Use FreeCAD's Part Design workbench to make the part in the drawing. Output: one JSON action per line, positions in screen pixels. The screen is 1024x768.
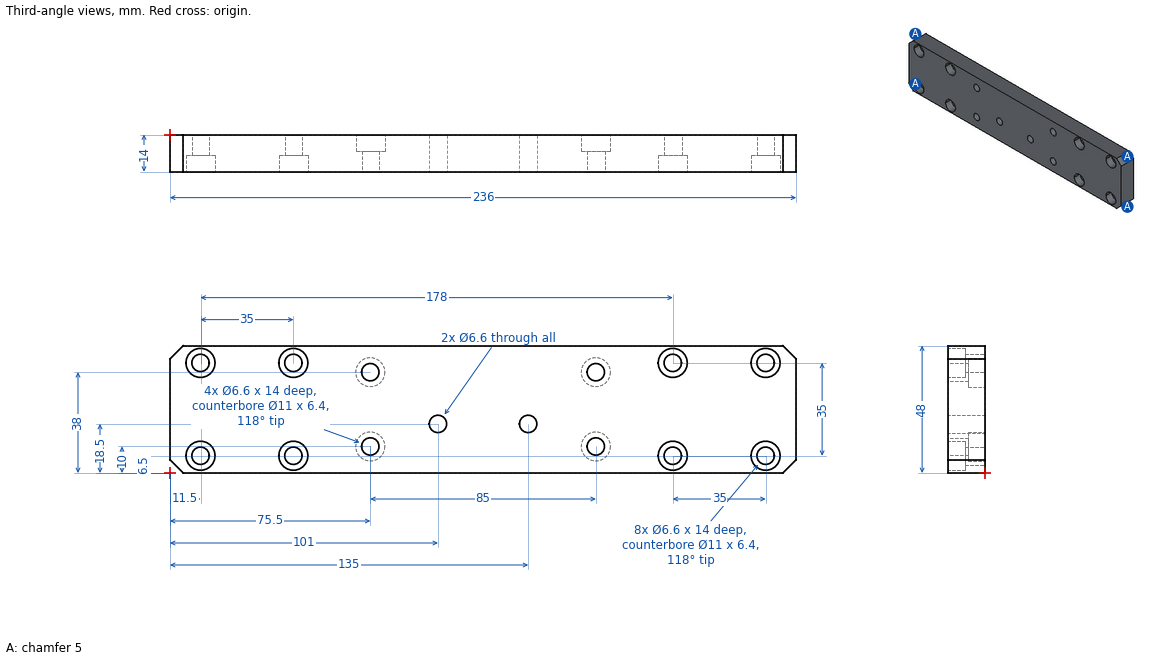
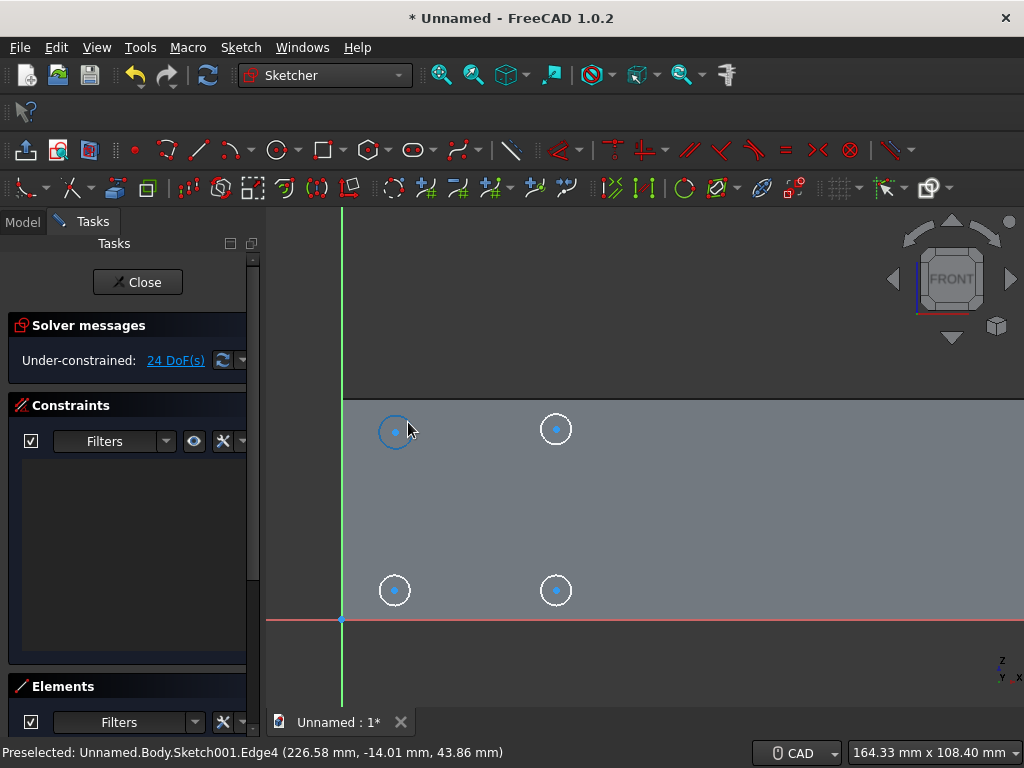
{"action": "left_click", "coordinate": [408, 420]}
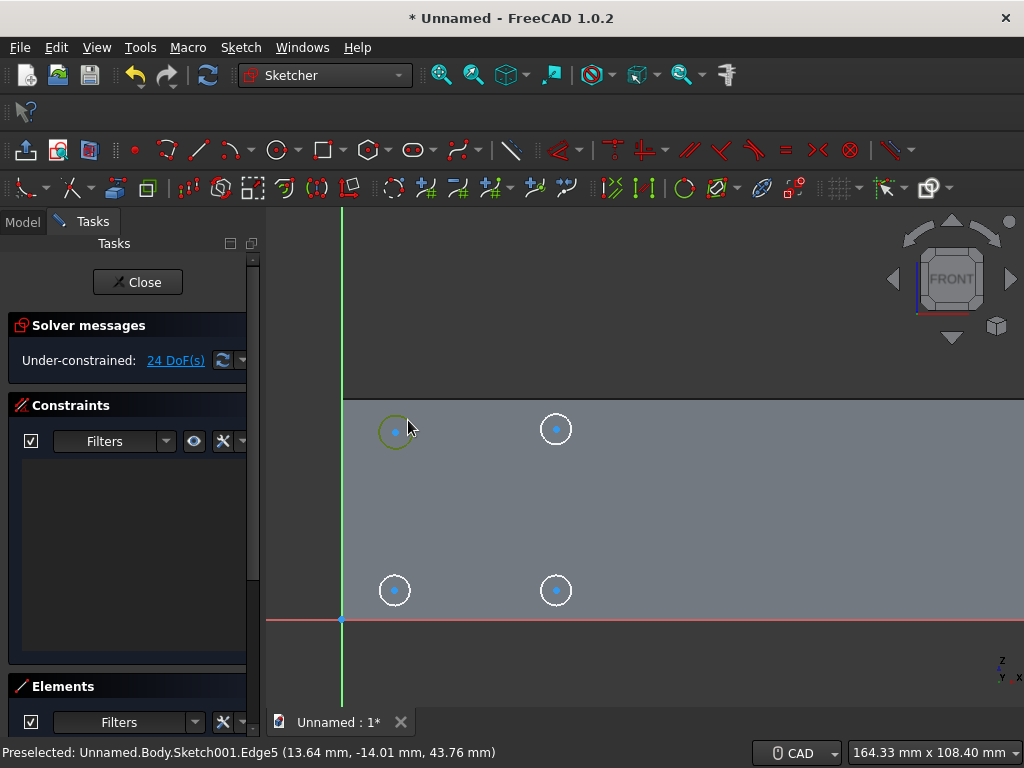
{"action": "left_click", "coordinate": [567, 419]}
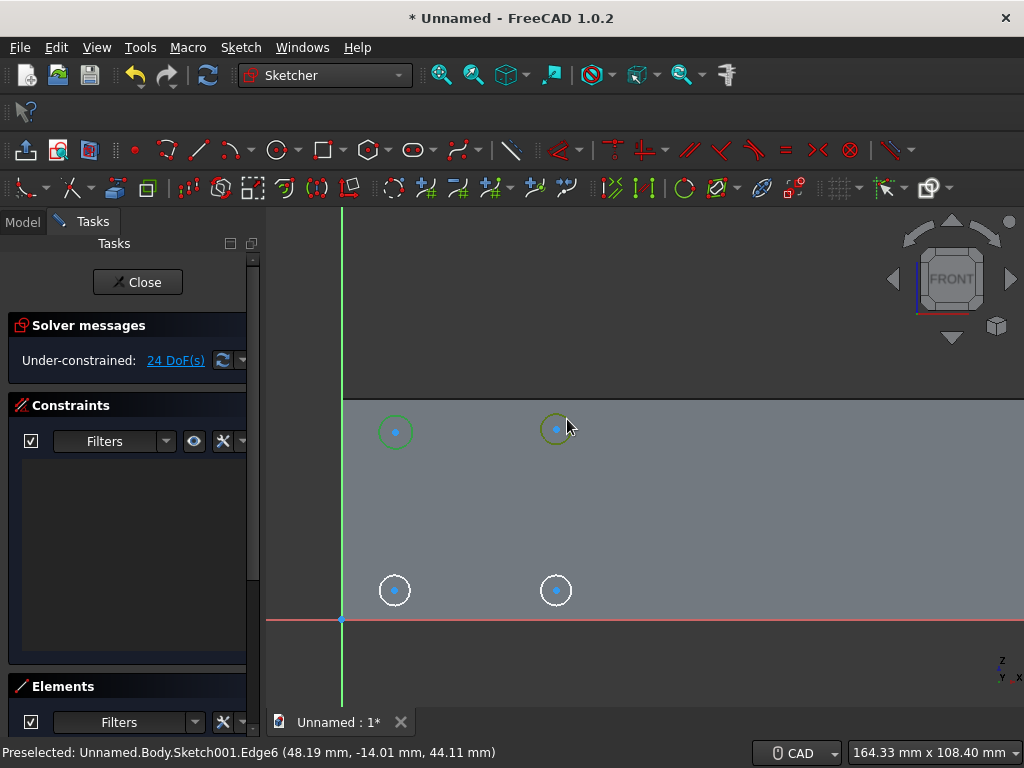
{"action": "left_click", "coordinate": [567, 580]}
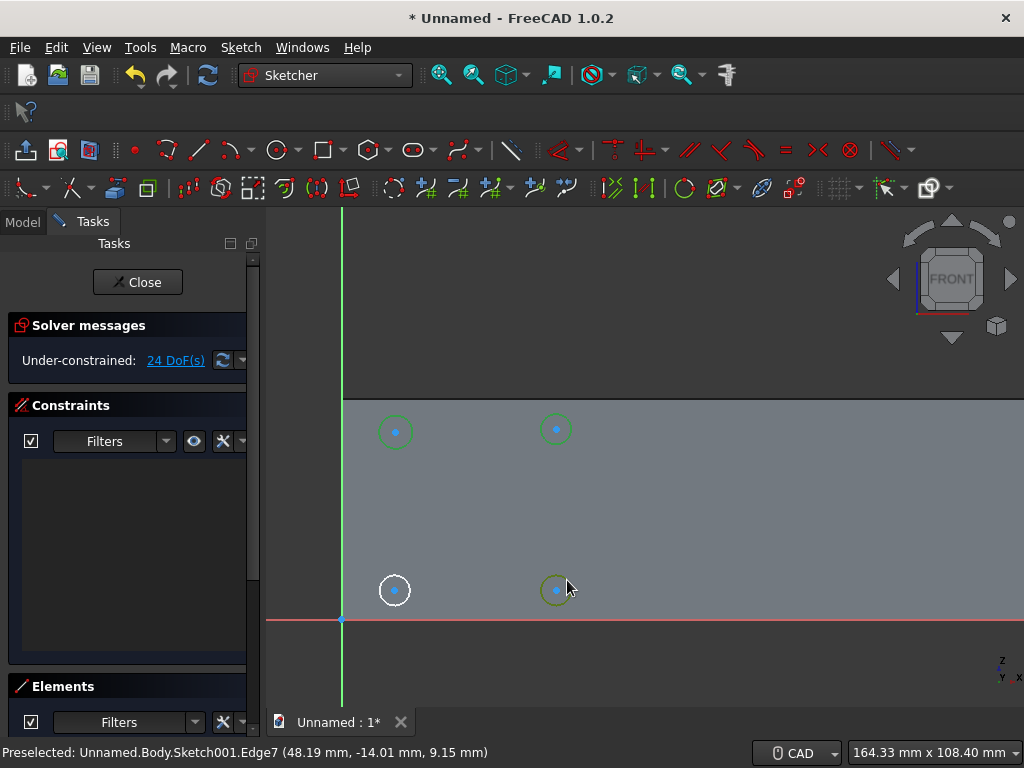
{"action": "left_click", "coordinate": [405, 580]}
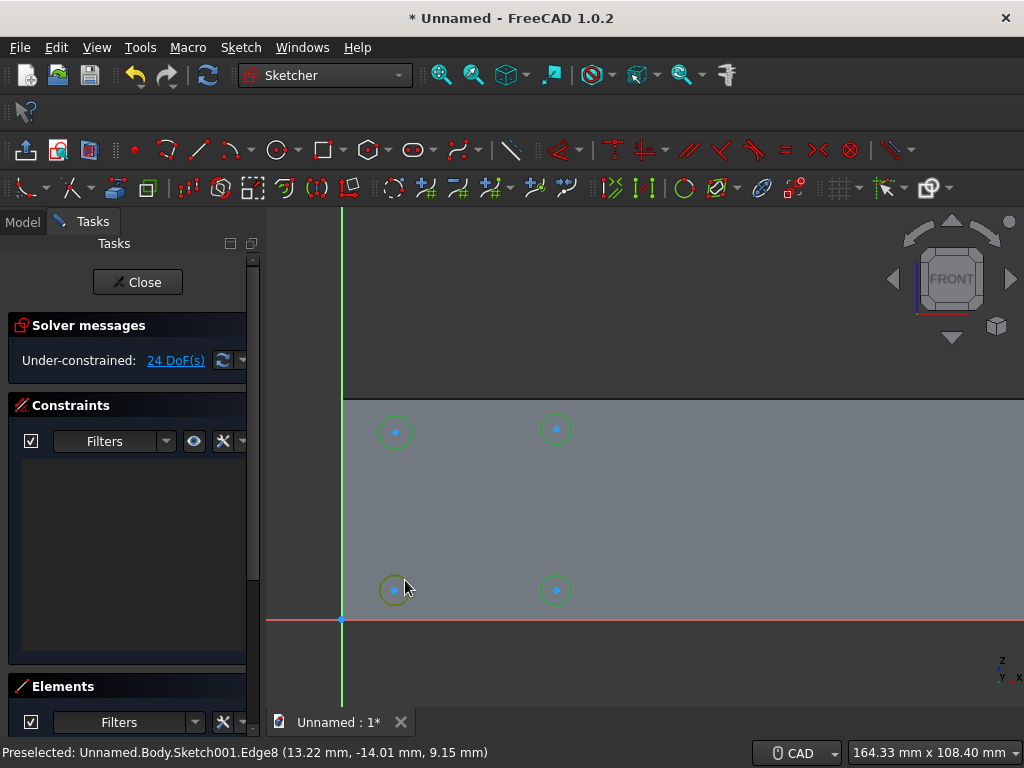
{"action": "left_click", "coordinate": [786, 150]}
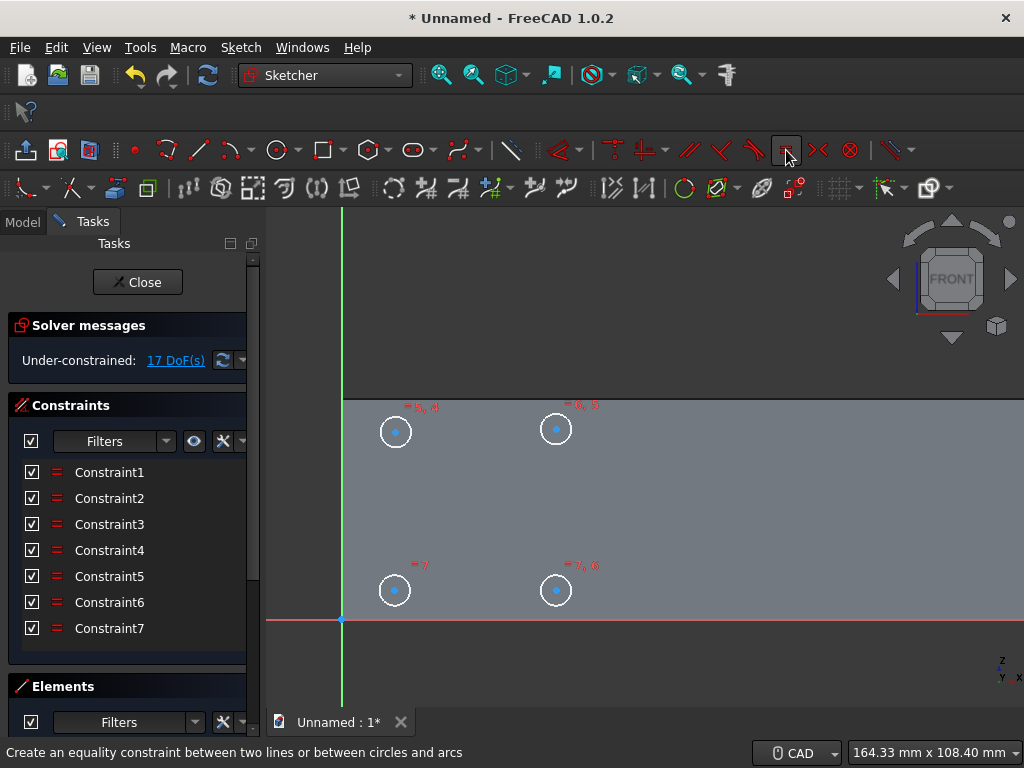
{"action": "scroll", "coordinate": [407, 422], "scroll_direction": "down", "scroll_amount": 5}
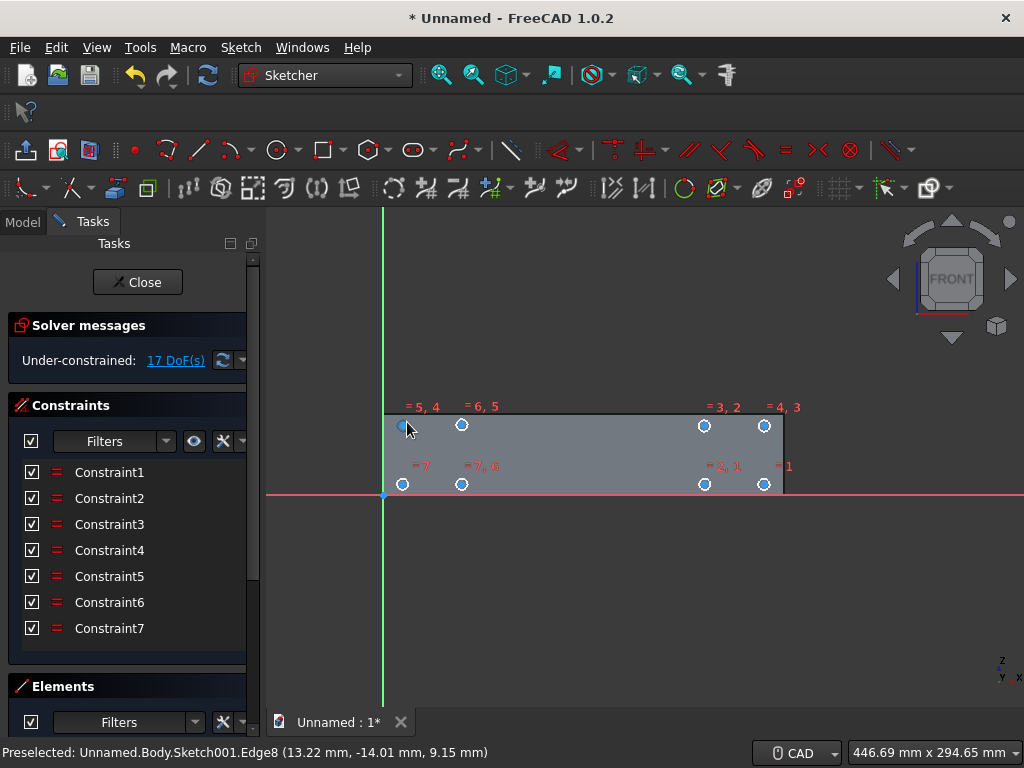
{"action": "left_click", "coordinate": [764, 484]}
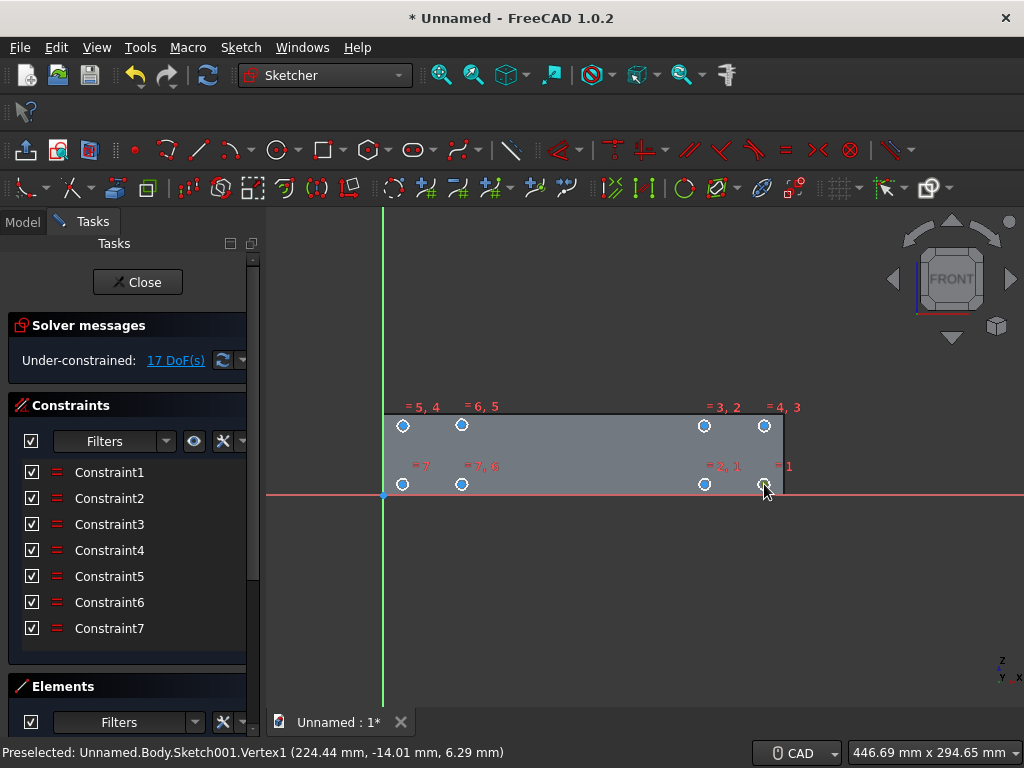
{"action": "left_click", "coordinate": [705, 484]}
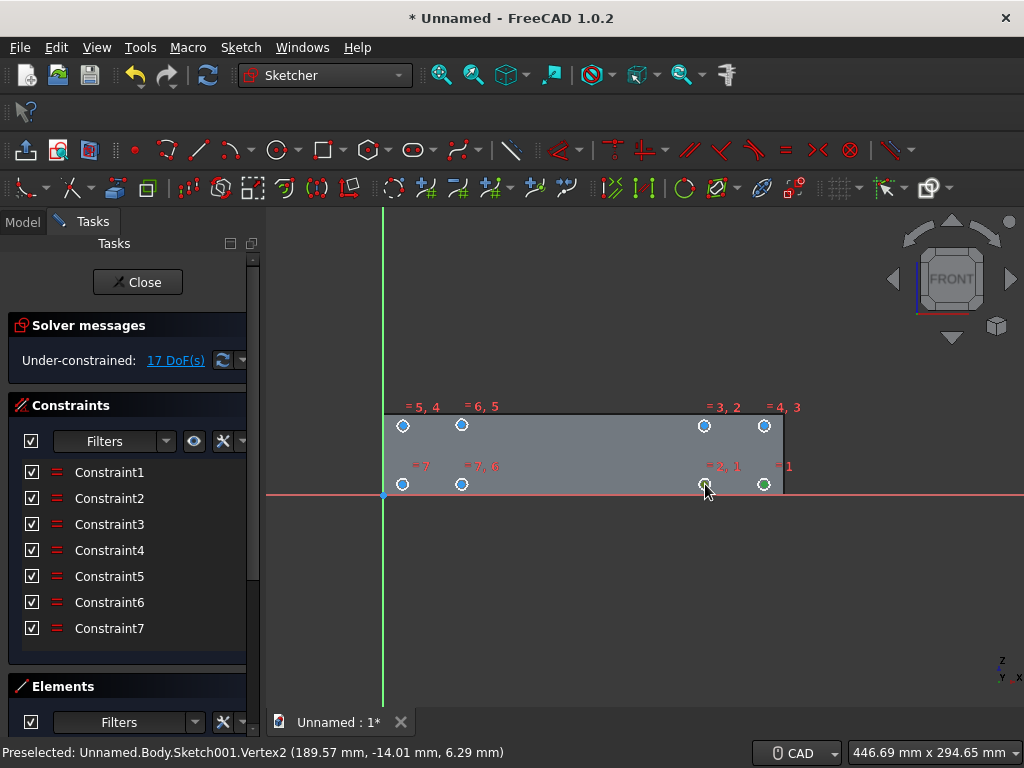
{"action": "left_click", "coordinate": [668, 150]}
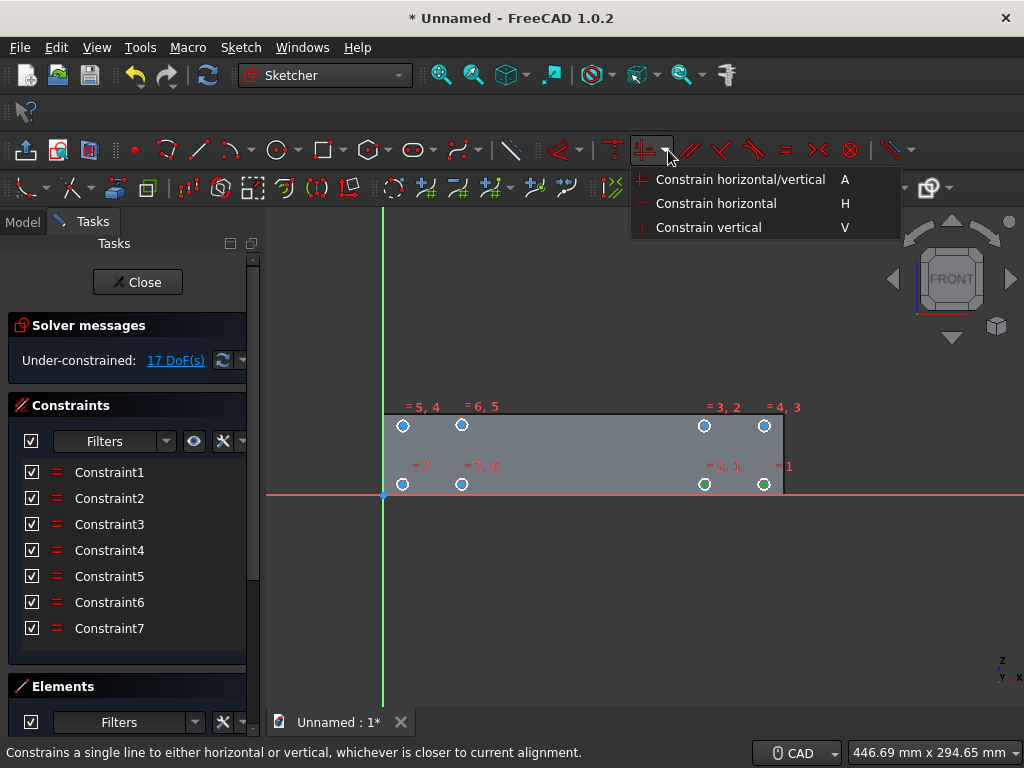
{"action": "left_click", "coordinate": [766, 203]}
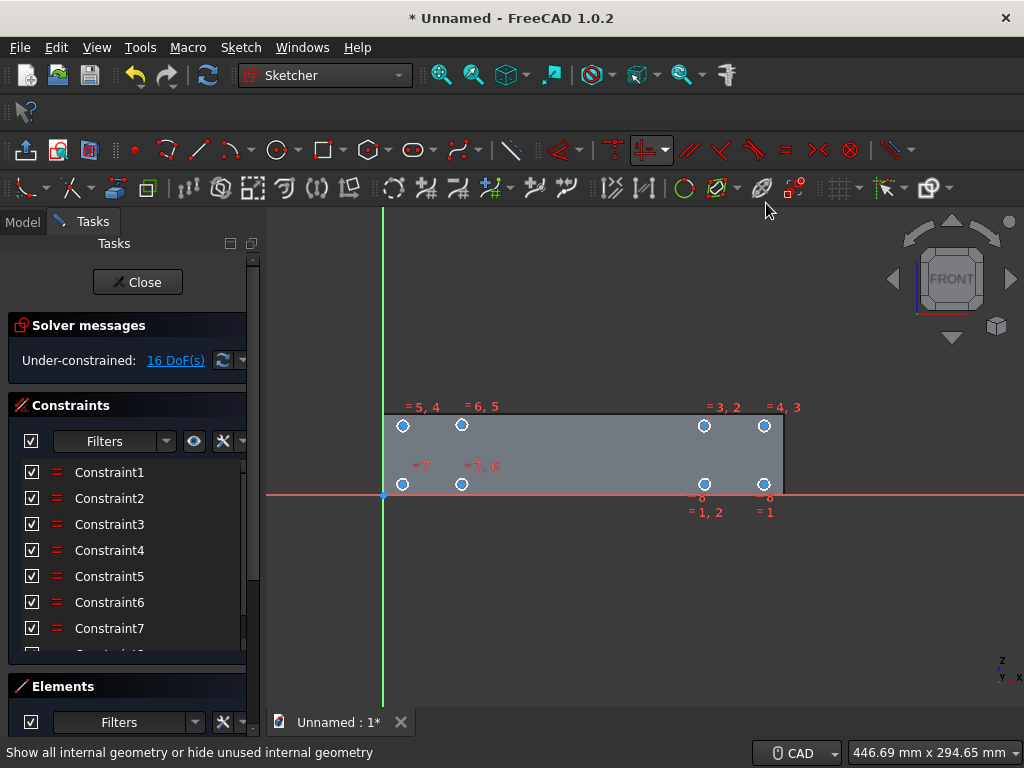
{"action": "left_click", "coordinate": [705, 484]}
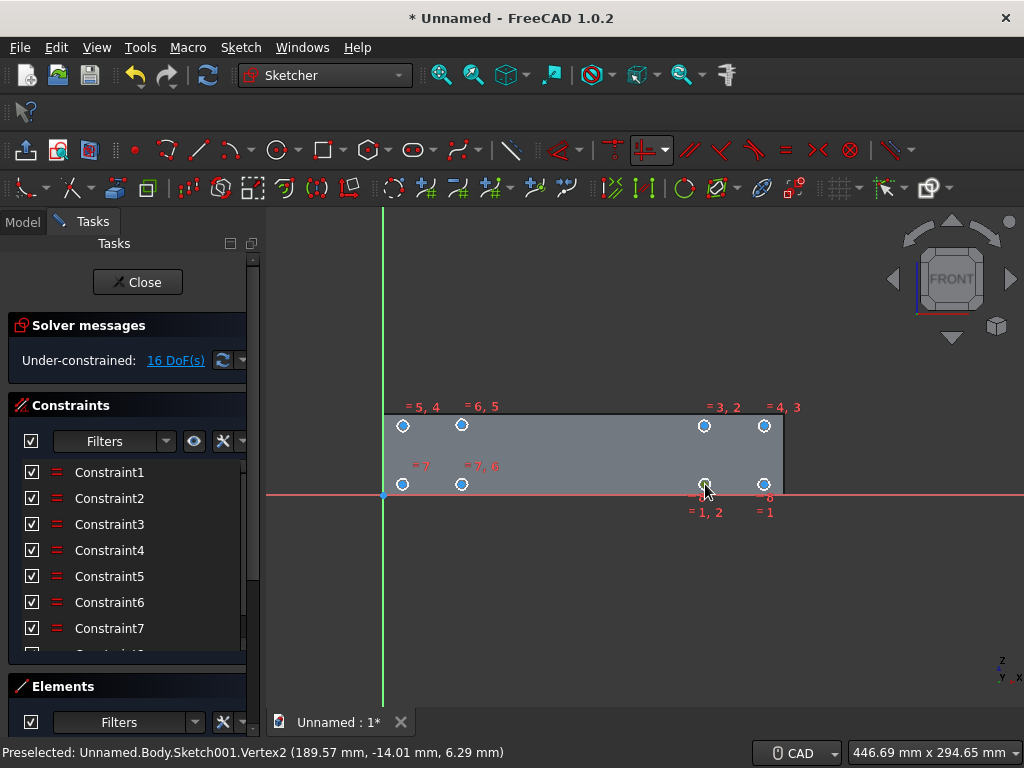
{"action": "left_click", "coordinate": [704, 426]}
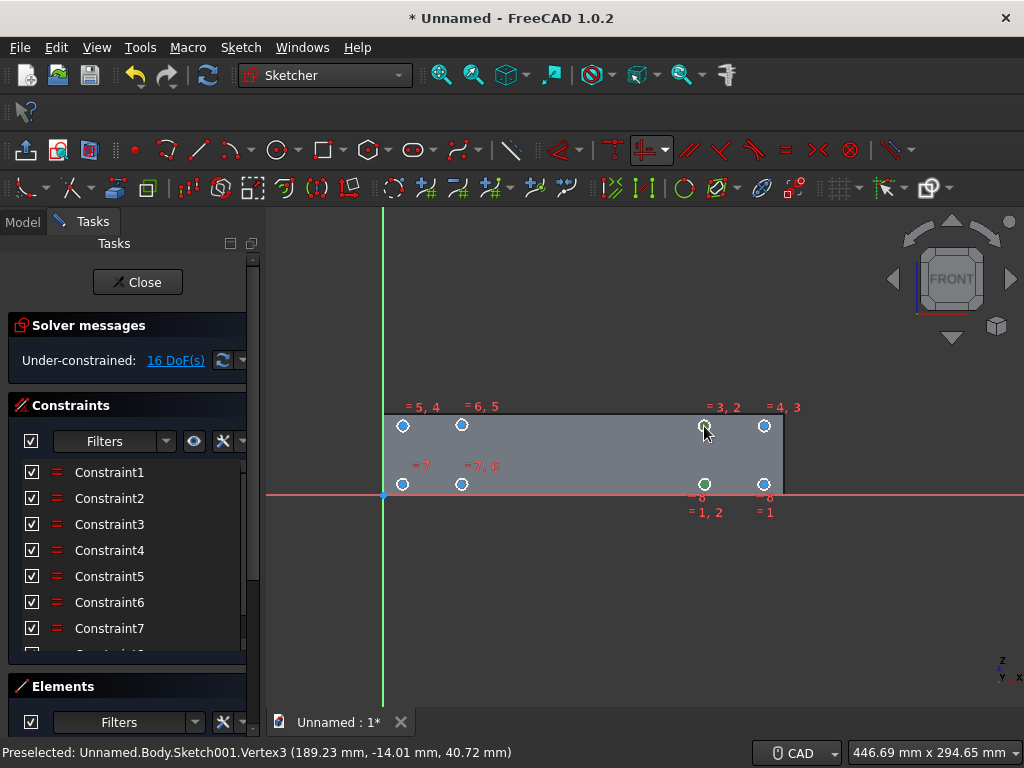
{"action": "left_click", "coordinate": [668, 150]}